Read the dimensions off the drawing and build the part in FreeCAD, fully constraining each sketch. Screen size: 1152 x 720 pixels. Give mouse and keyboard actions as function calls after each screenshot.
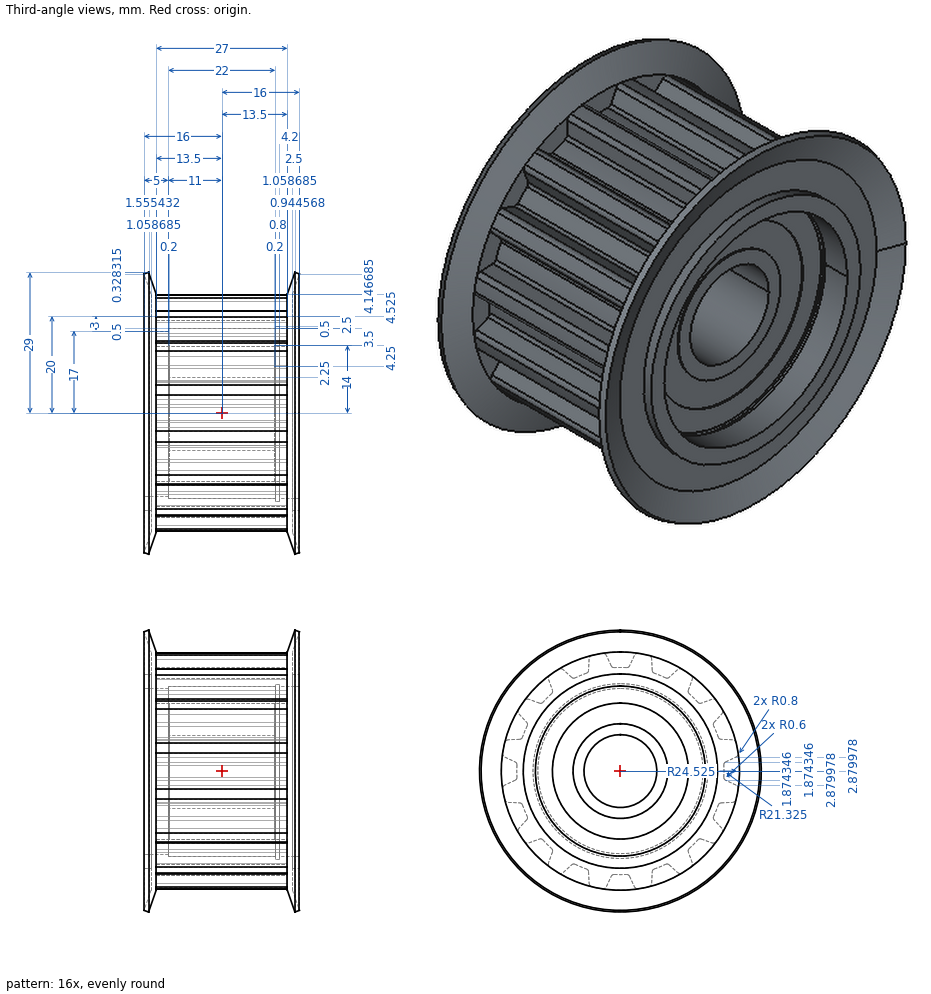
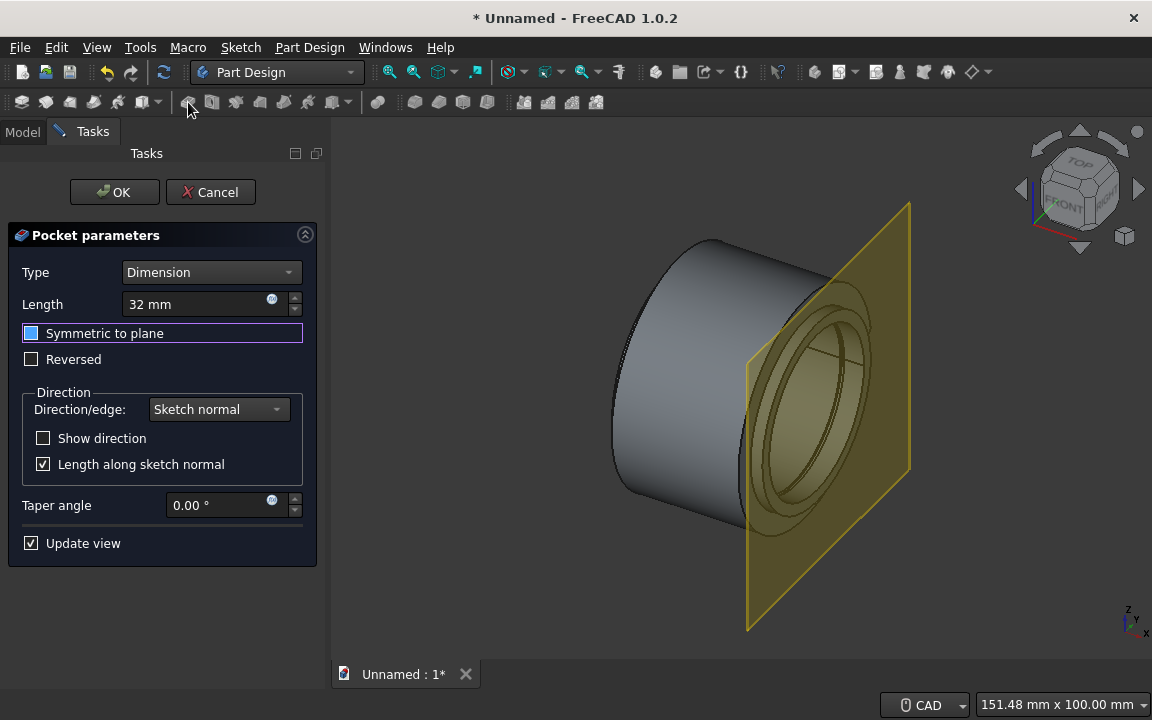
click(115, 192)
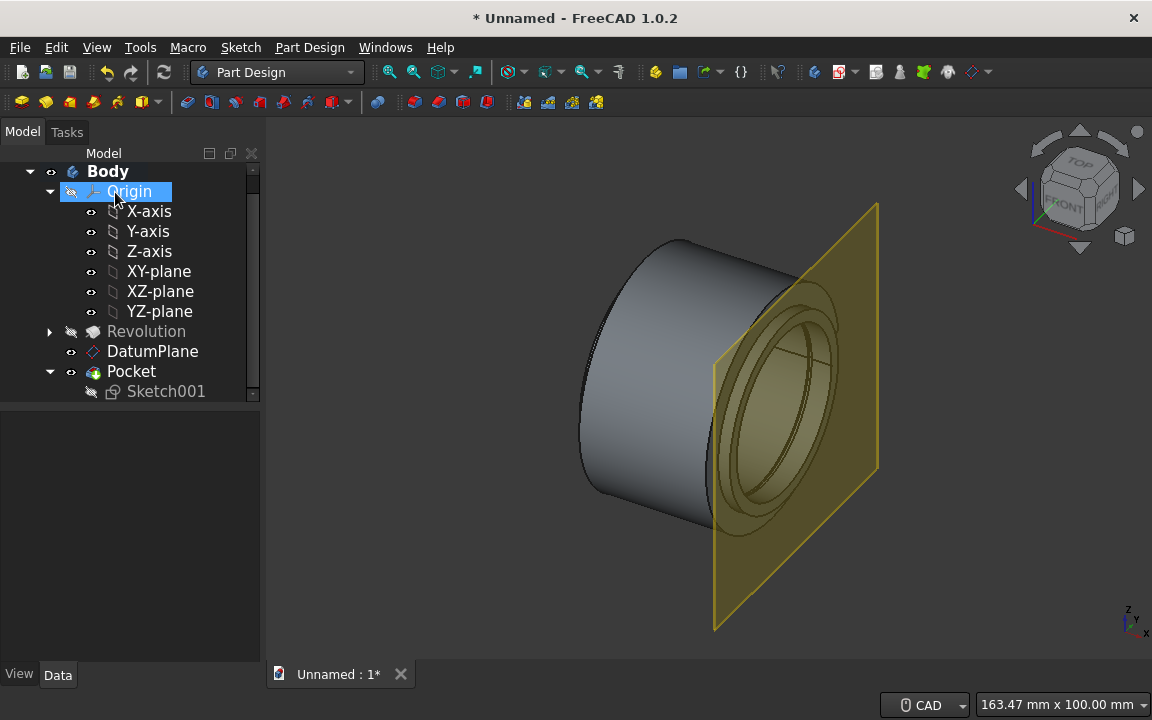
click(116, 352)
key(space)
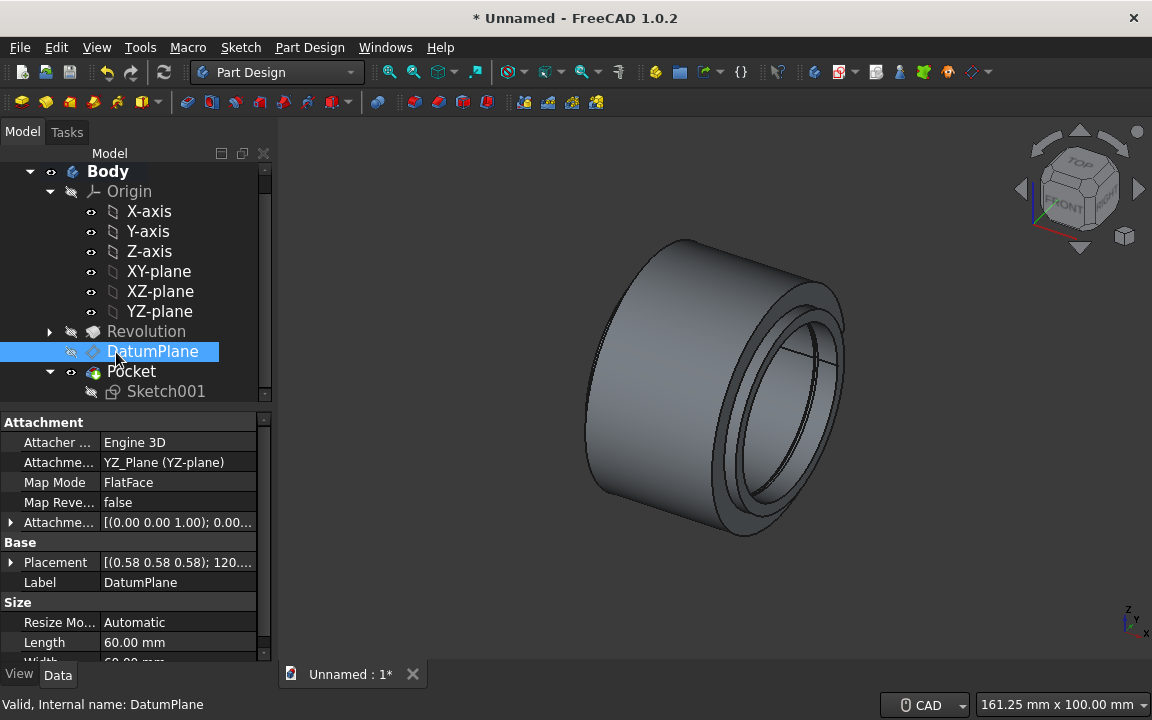
click(116, 372)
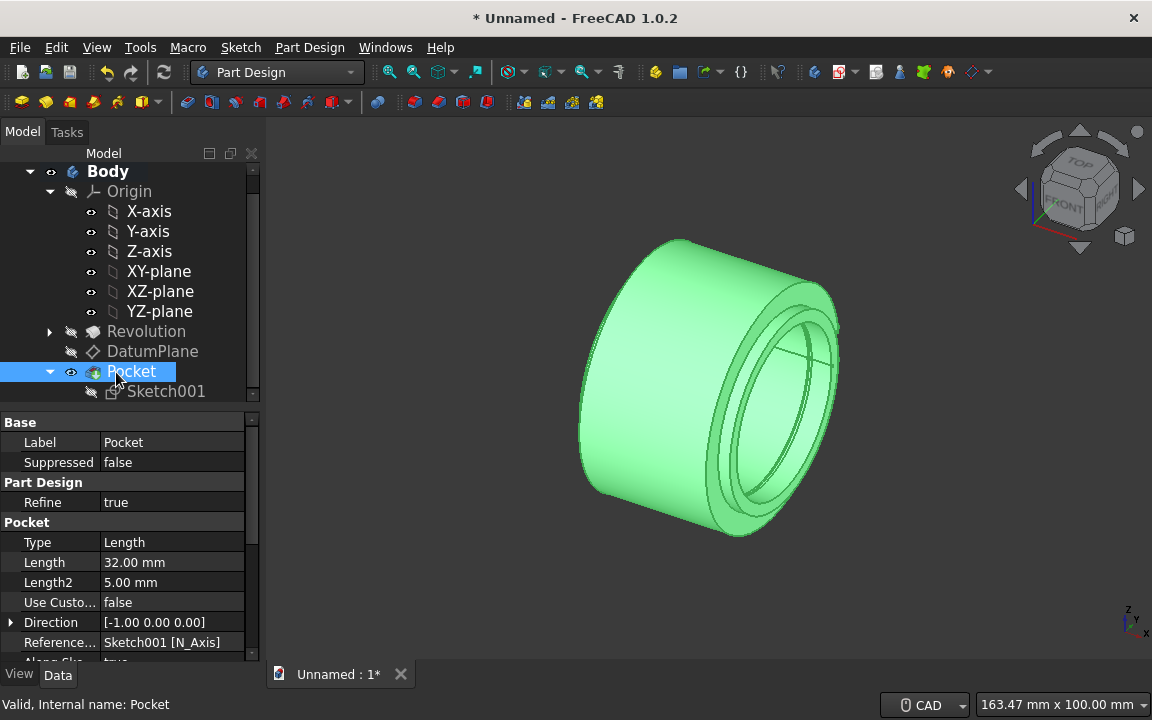
click(572, 102)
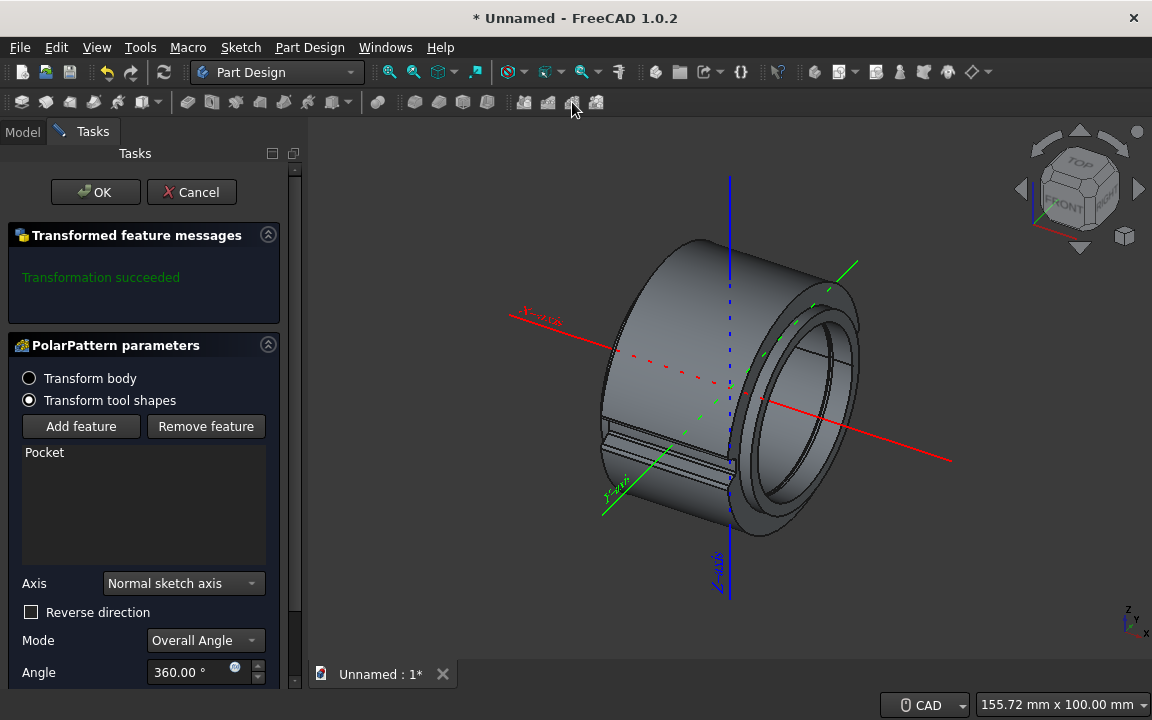
click(184, 584)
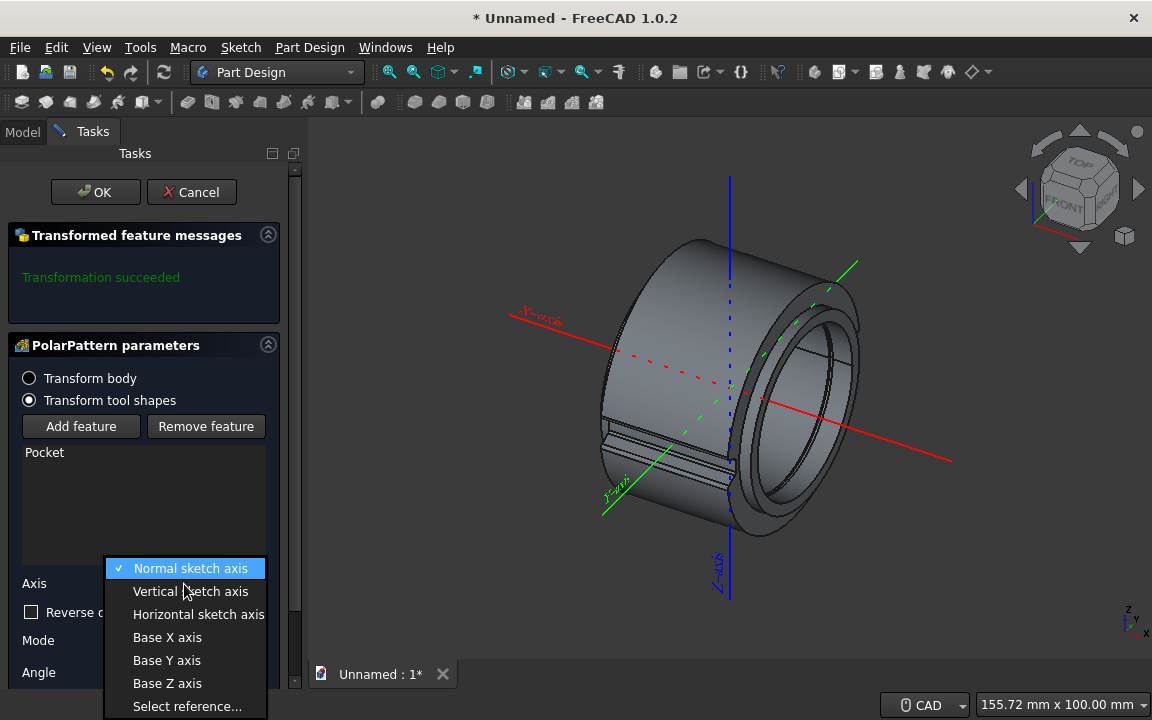
click(184, 638)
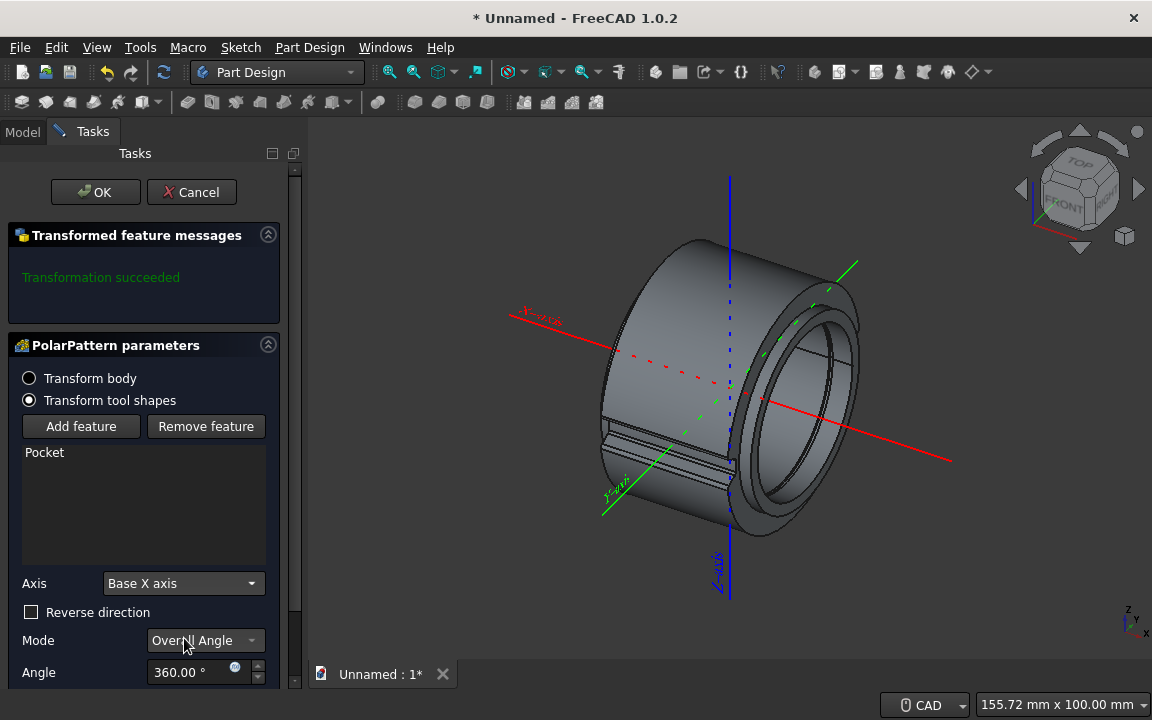
scroll(295, 426, down, 2)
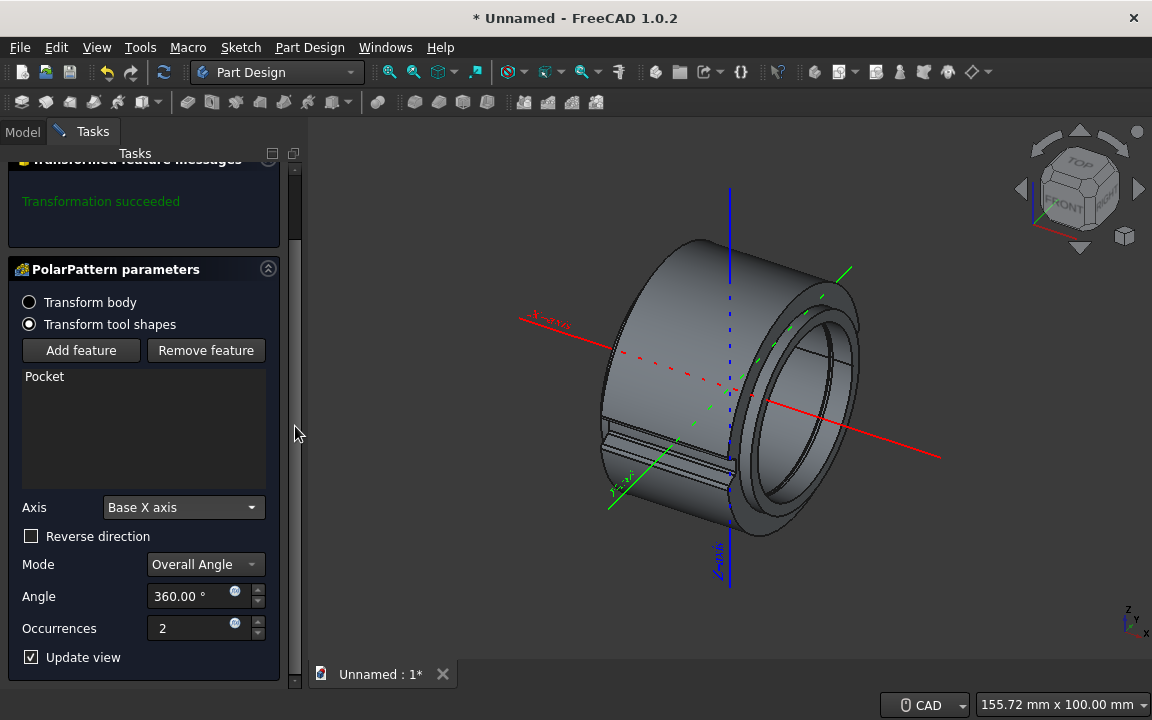
triple_click(198, 628)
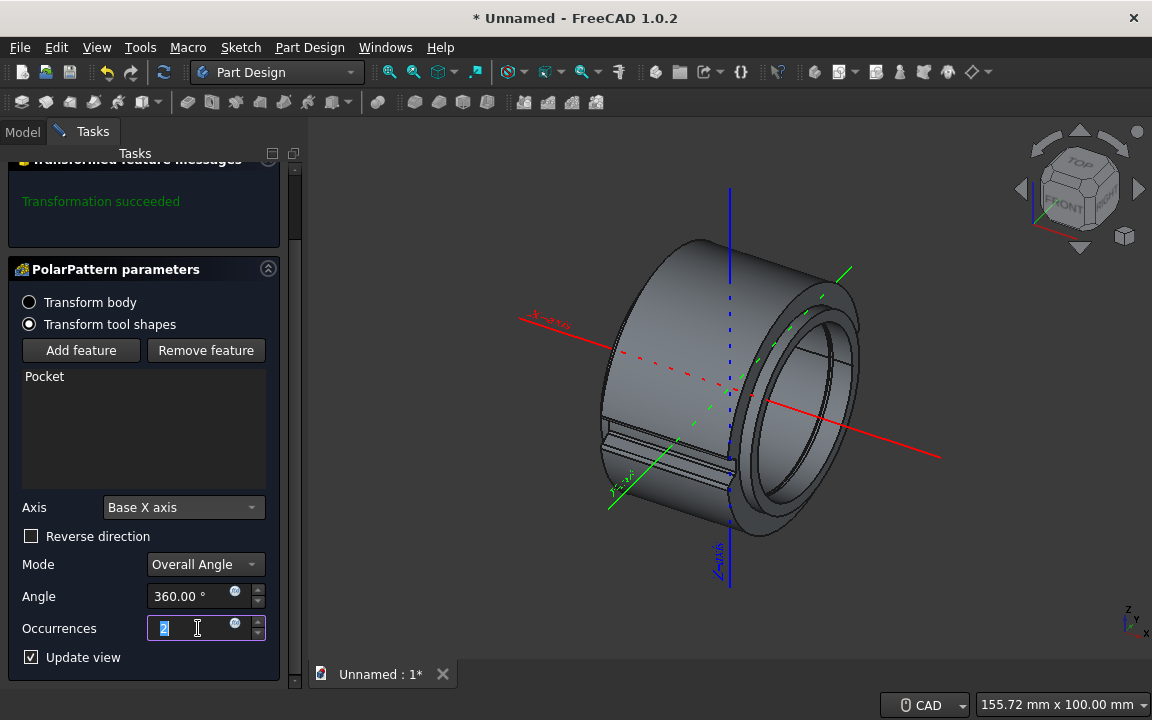
text(16)
key(Tab)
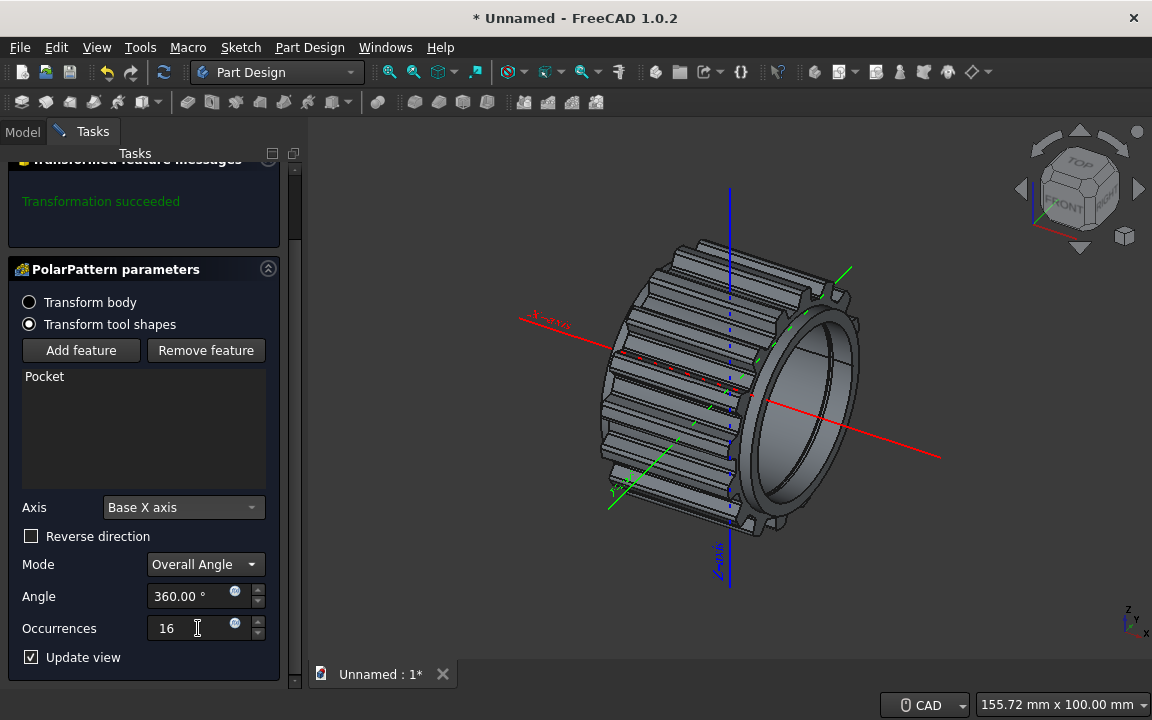
scroll(295, 426, up, 3)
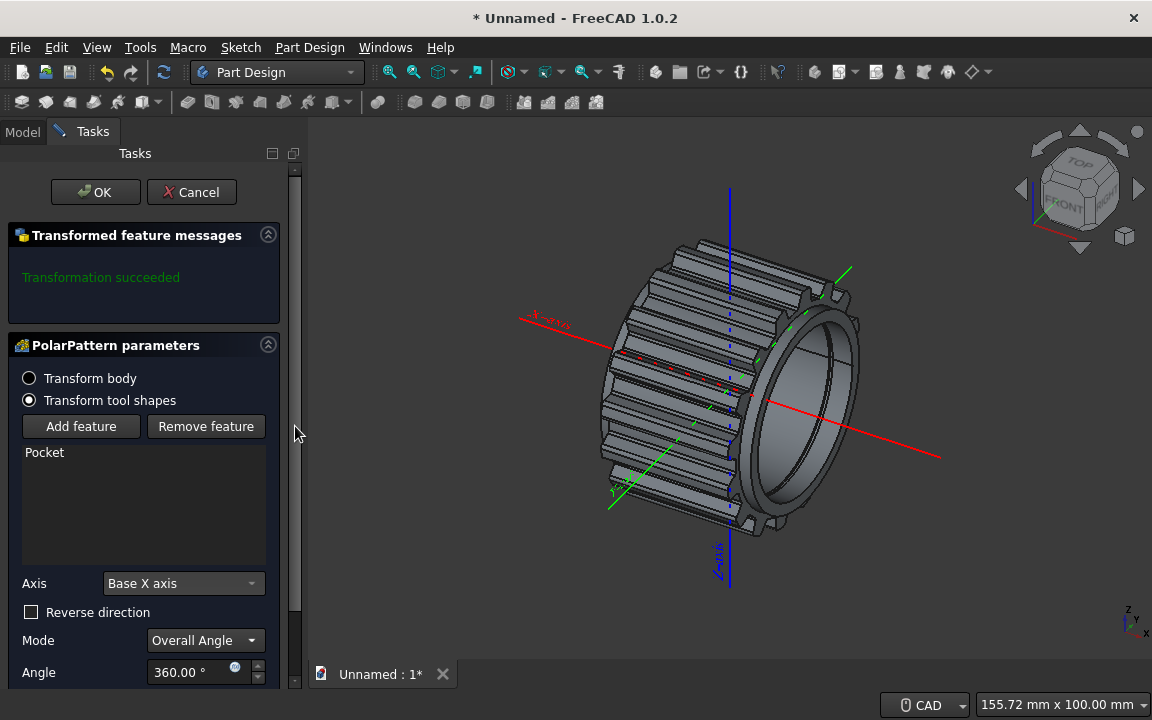
click(96, 192)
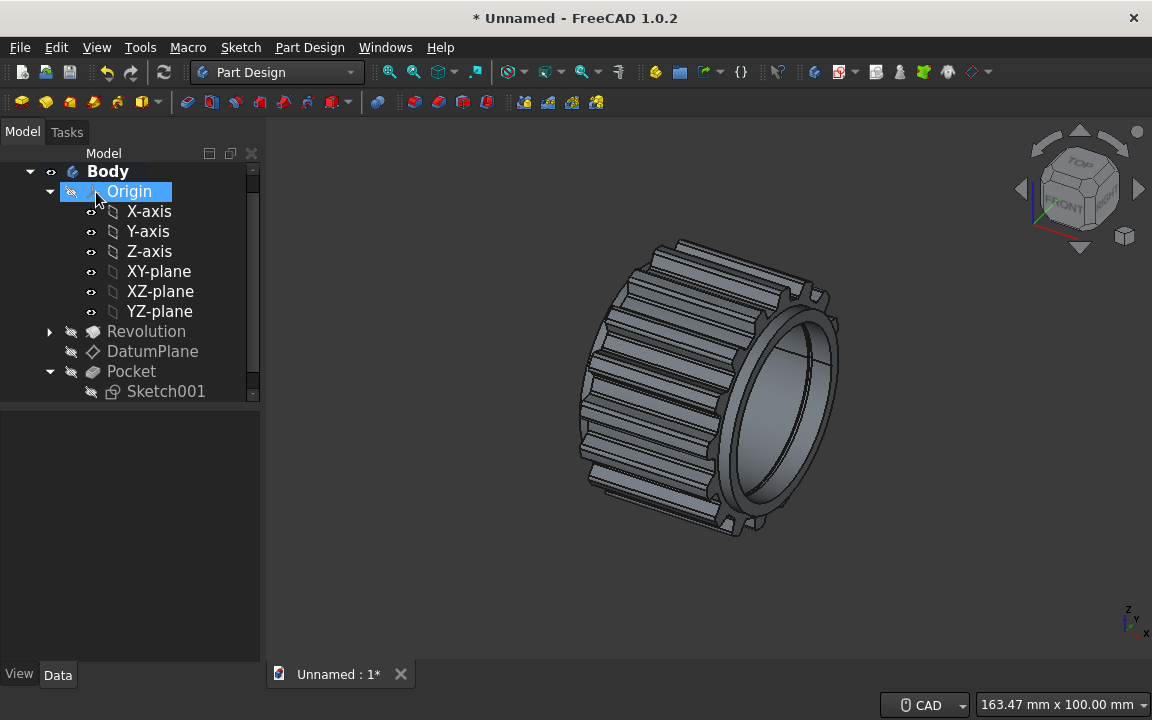
click(840, 72)